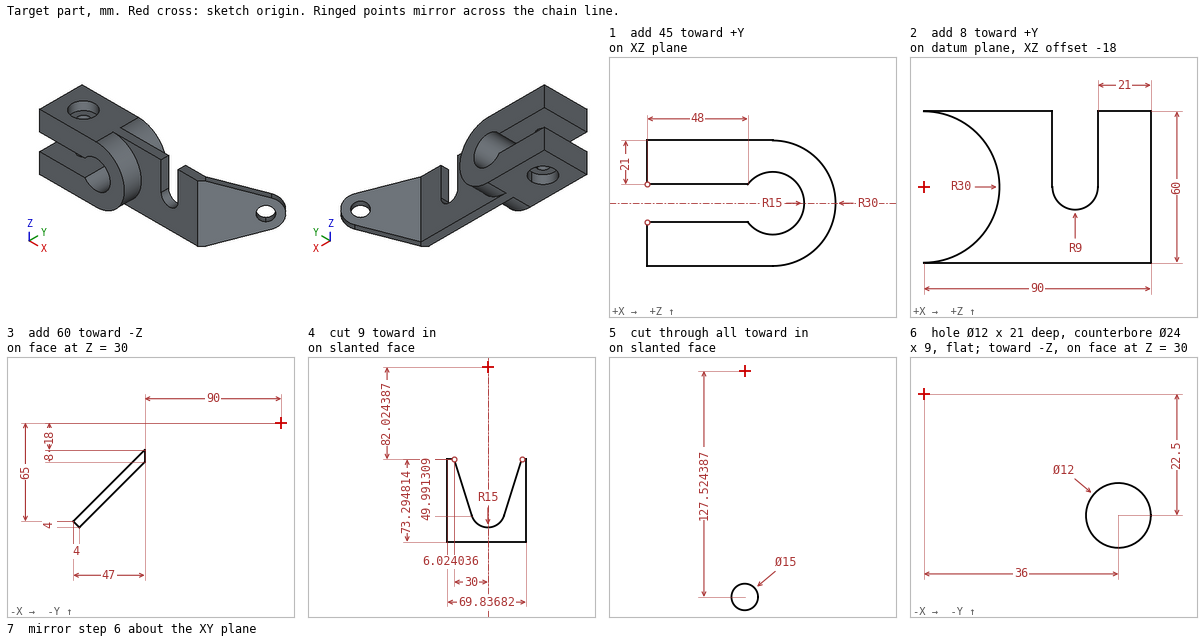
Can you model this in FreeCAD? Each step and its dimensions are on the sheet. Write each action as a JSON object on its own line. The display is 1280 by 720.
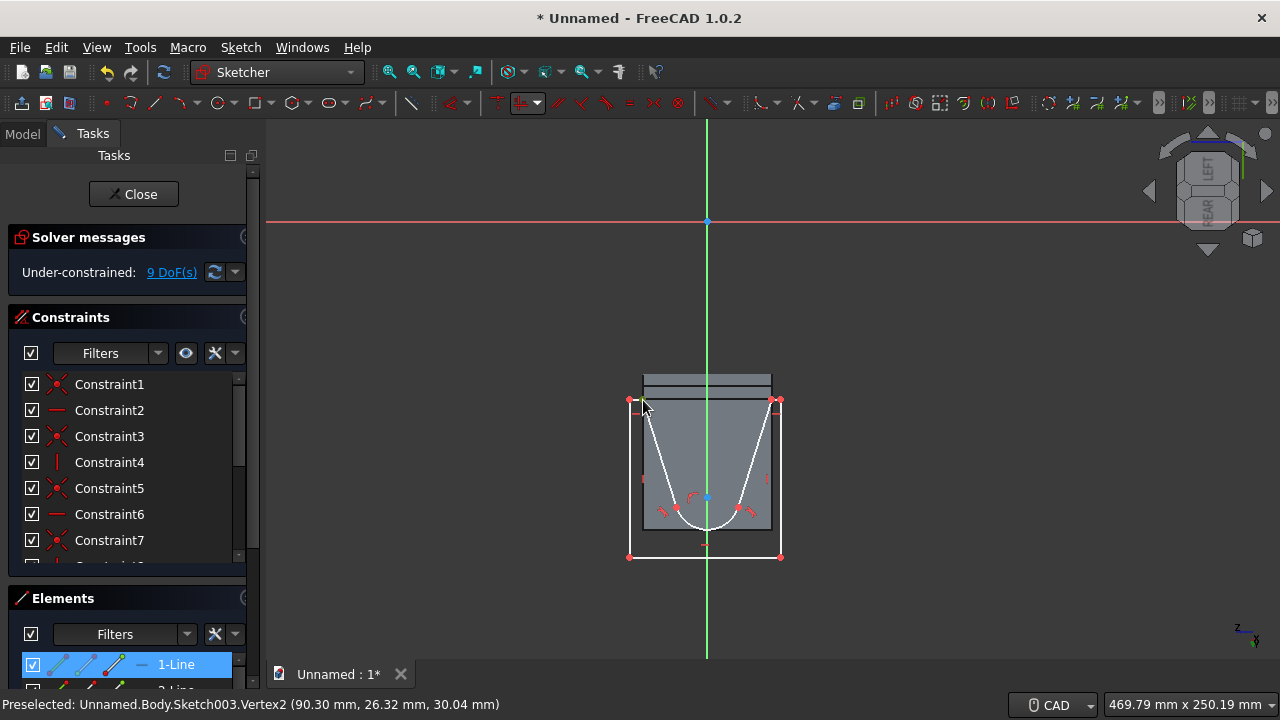
{"action": "scroll", "coordinate": [772, 400], "scroll_direction": "up", "scroll_amount": 2}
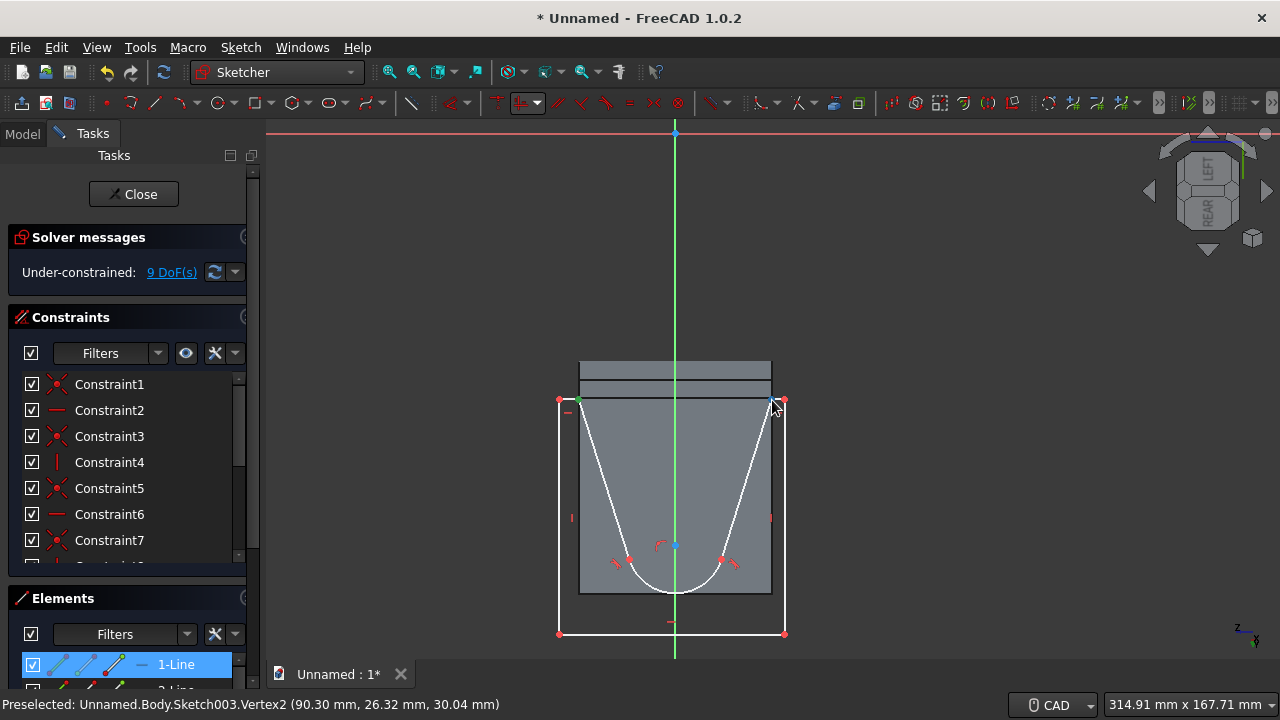
{"action": "left_click", "coordinate": [772, 399]}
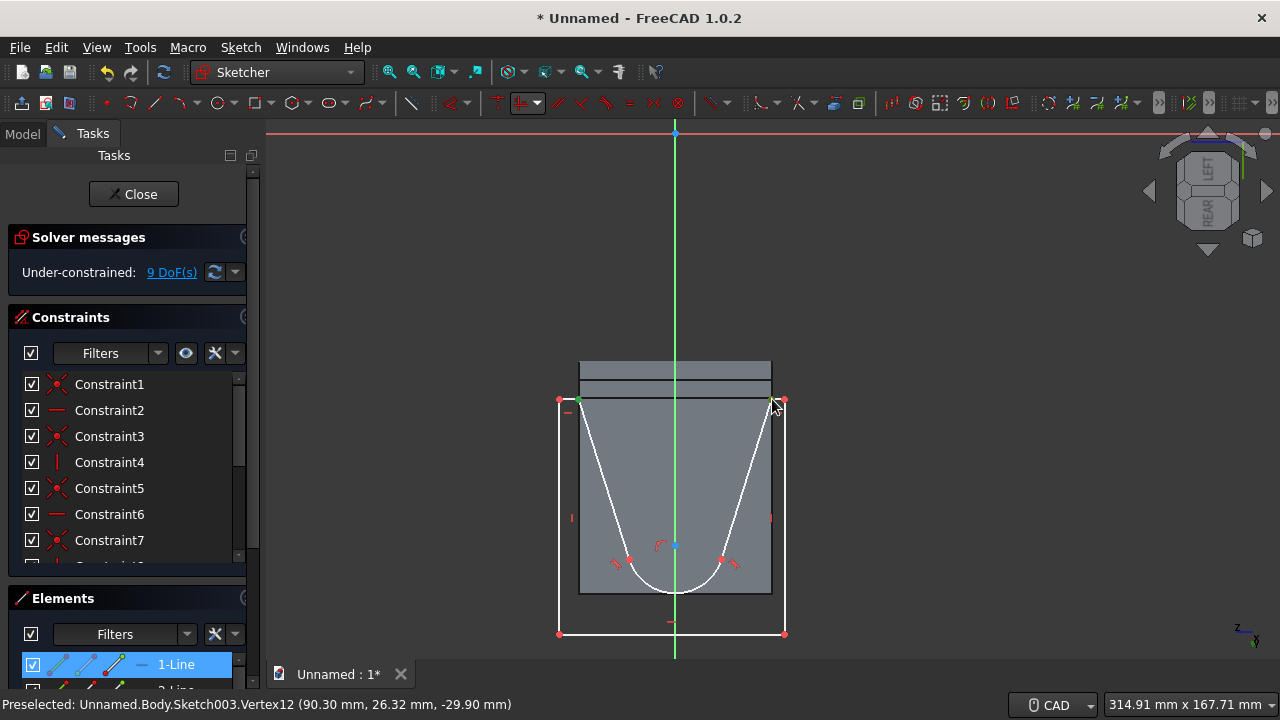
{"action": "left_click", "coordinate": [675, 562]}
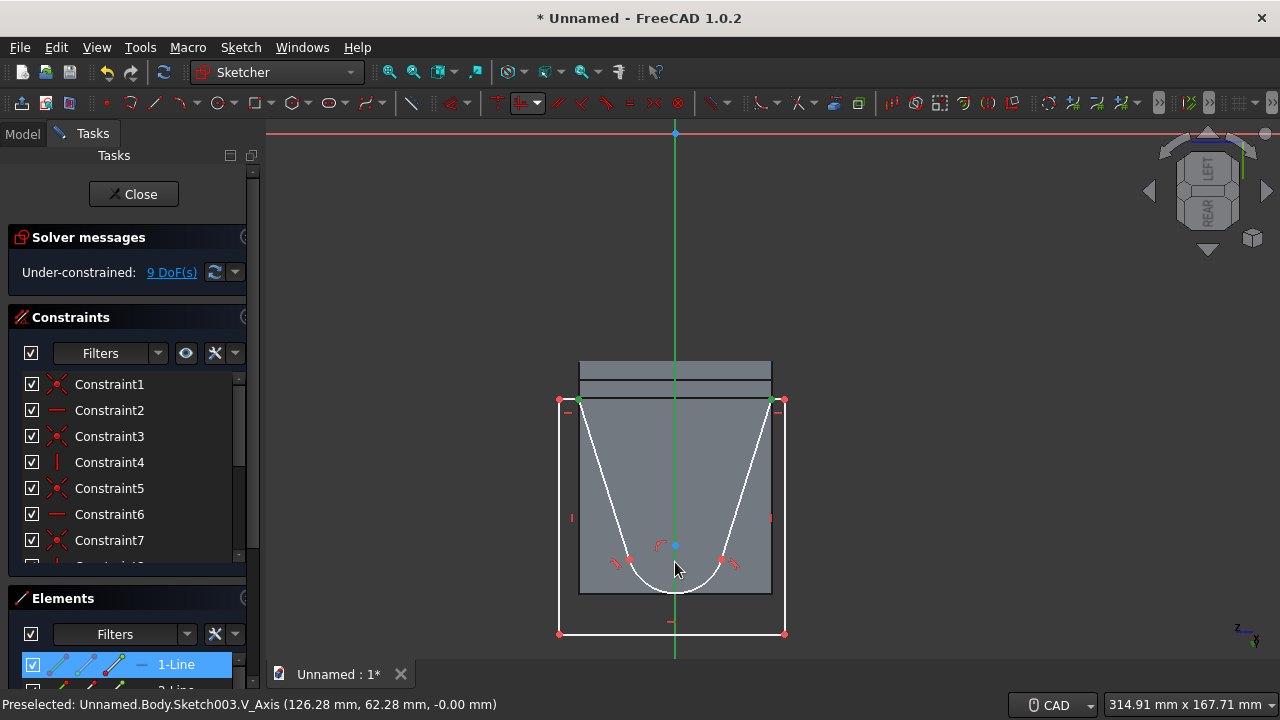
{"action": "left_click", "coordinate": [654, 104]}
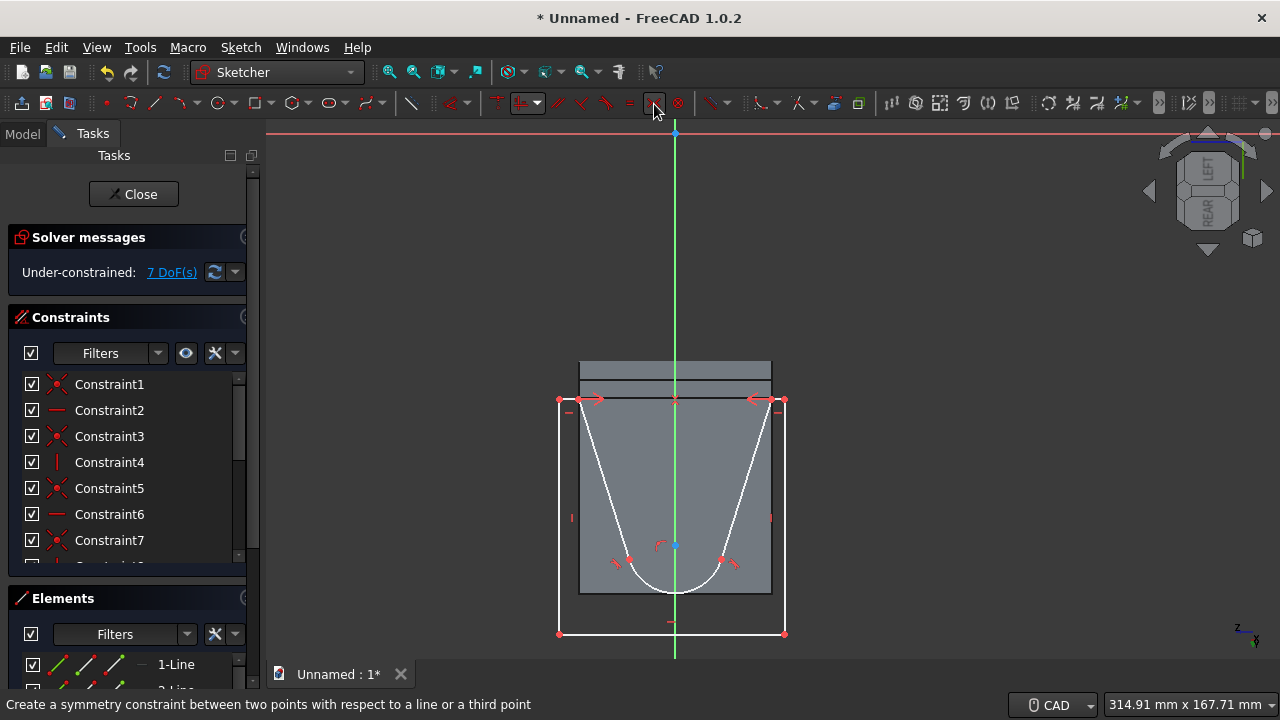
{"action": "left_click", "coordinate": [450, 104]}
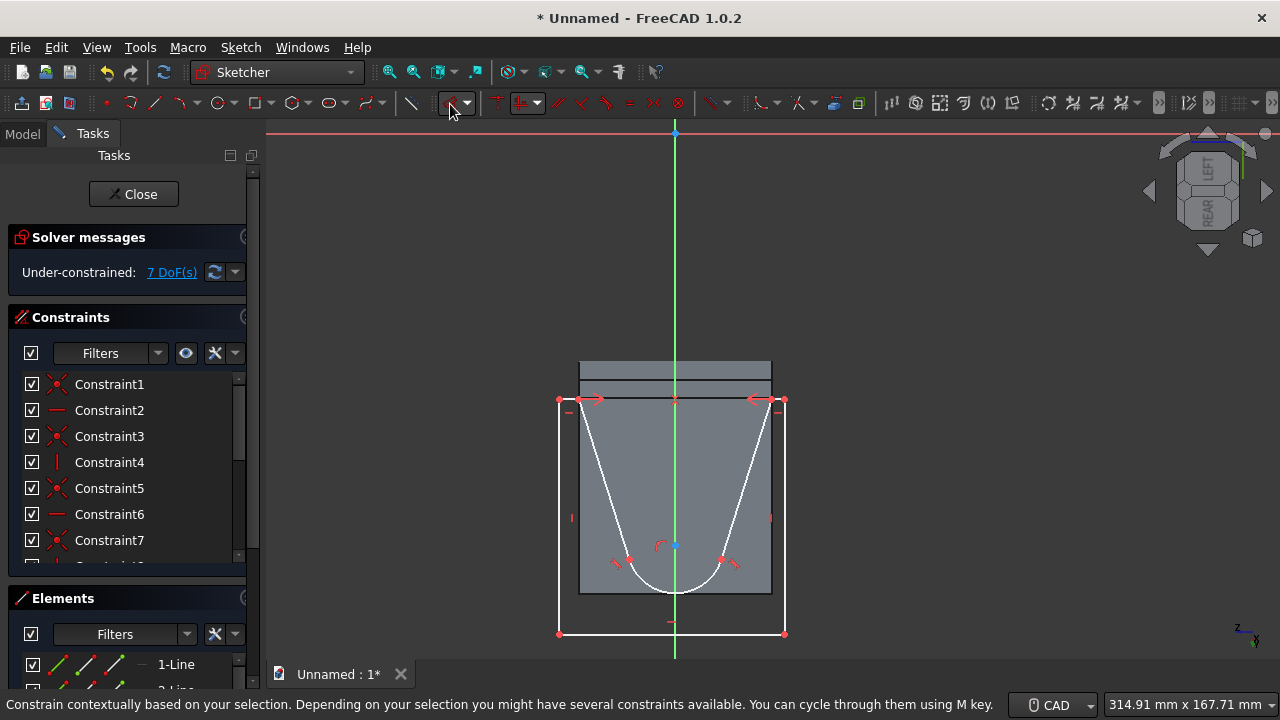
{"action": "left_click", "coordinate": [652, 587]}
{"action": "left_click", "coordinate": [636, 615]}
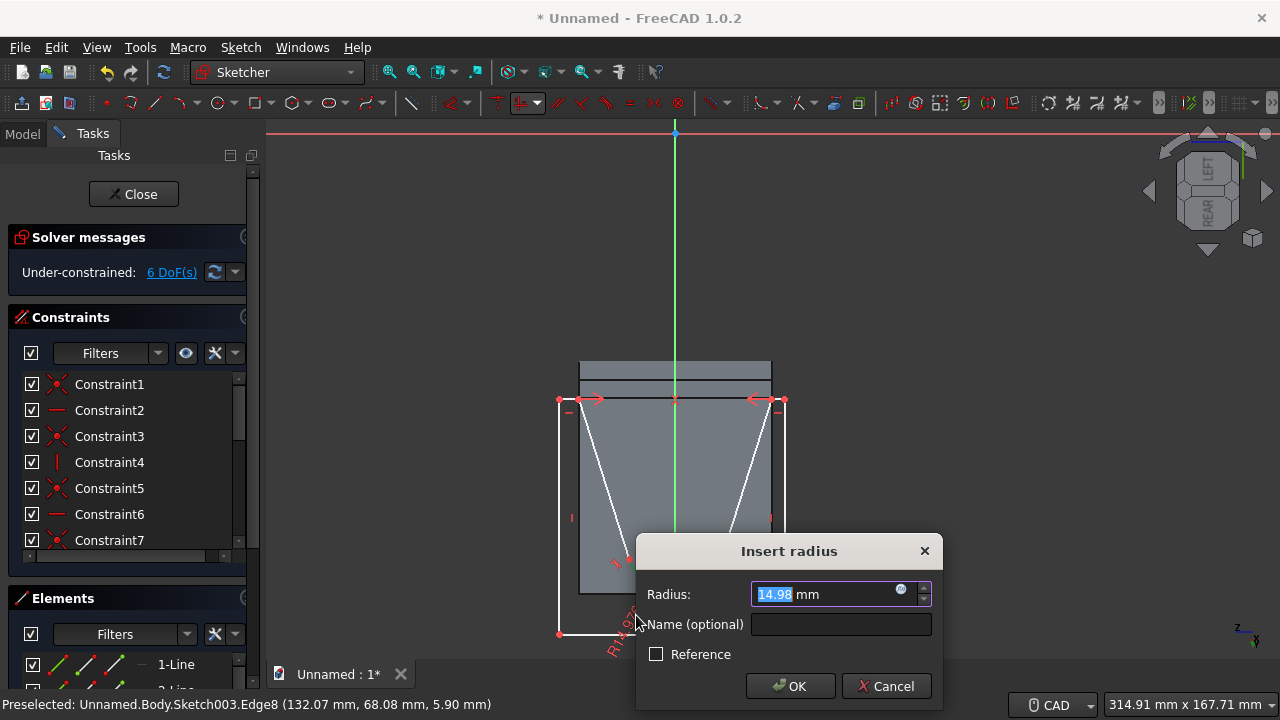
{"action": "type", "text": "15"}
{"action": "key", "text": "Return"}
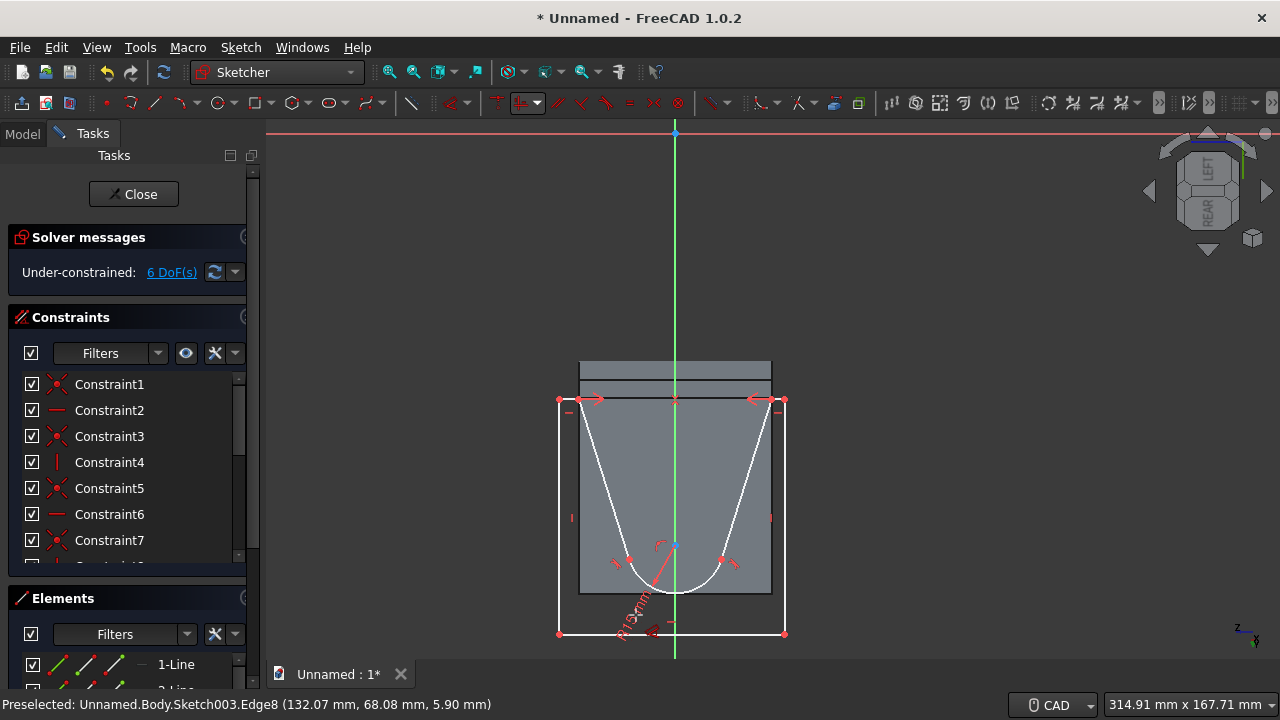
{"action": "left_click", "coordinate": [579, 399]}
{"action": "left_click", "coordinate": [627, 433]}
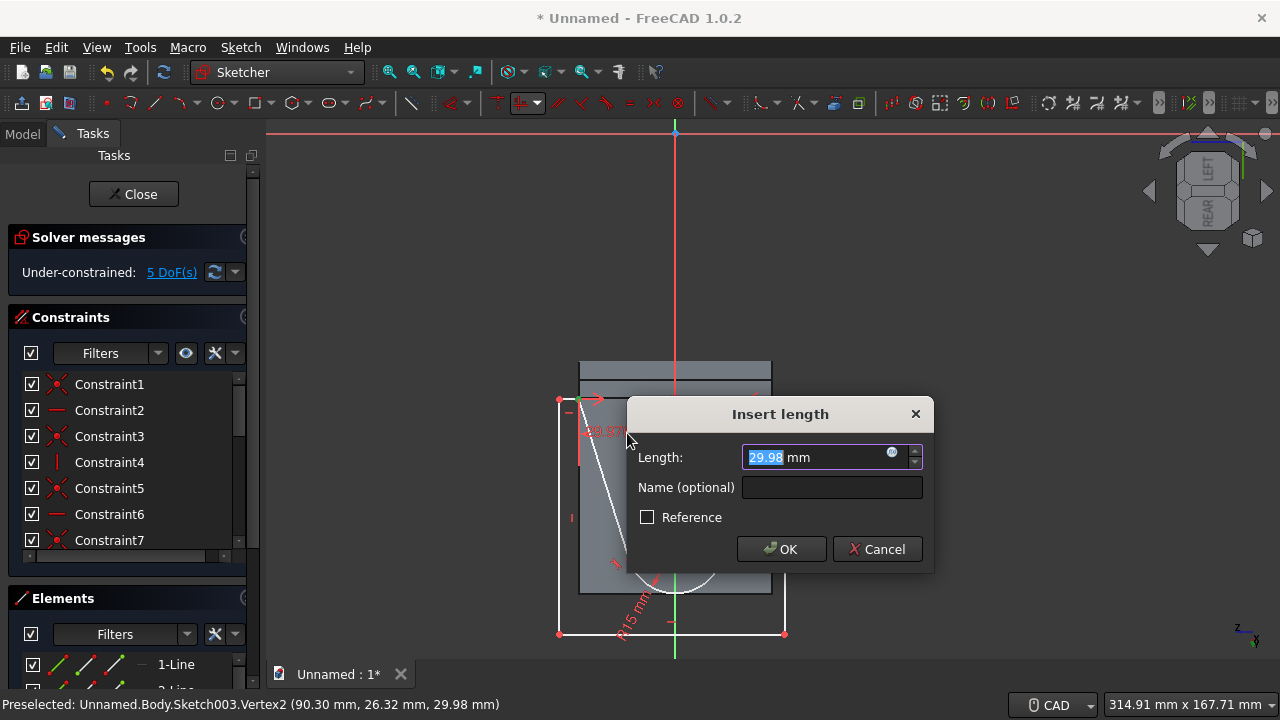
{"action": "type", "text": "30"}
{"action": "key", "text": "Return"}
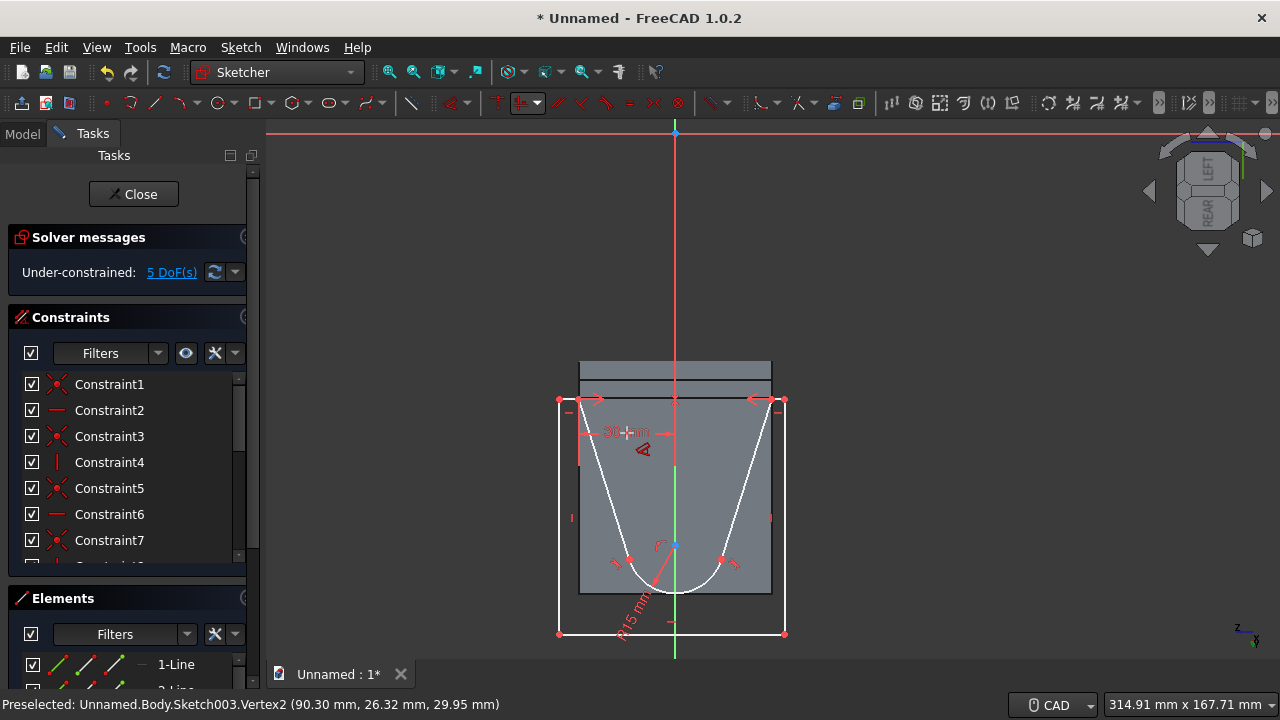
{"action": "scroll", "coordinate": [569, 399], "scroll_direction": "up", "scroll_amount": 4}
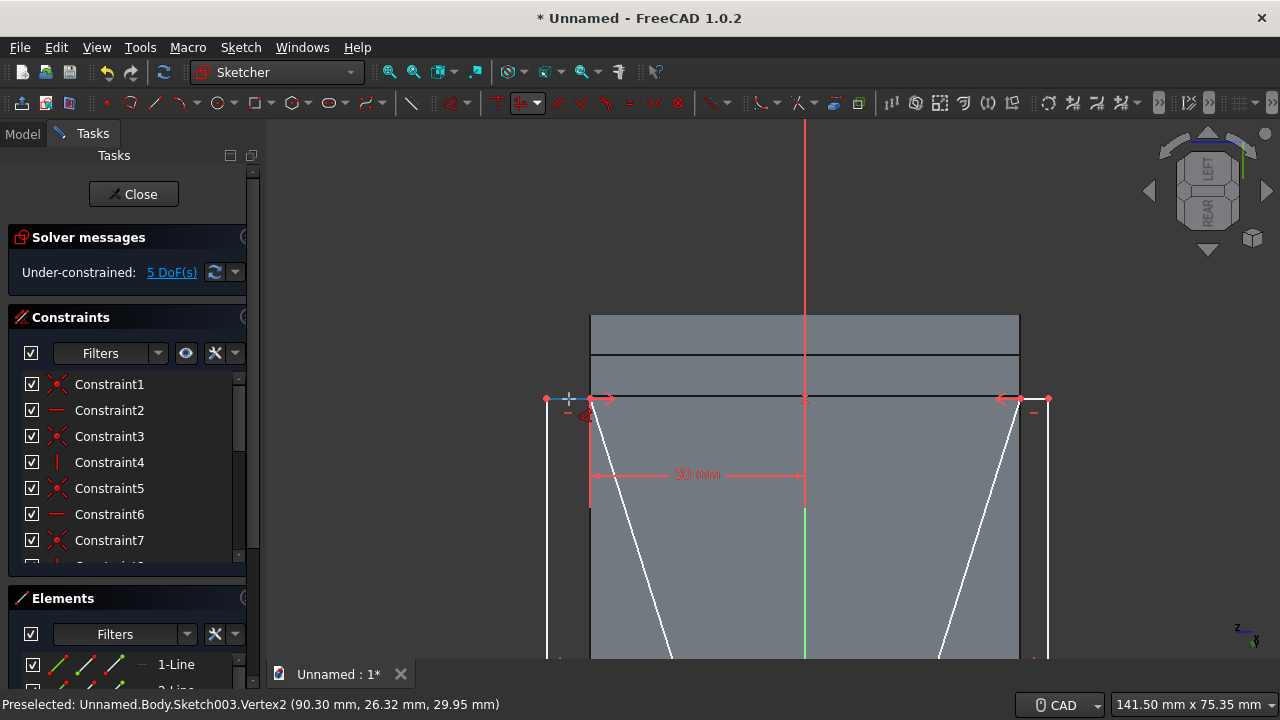
{"action": "left_click", "coordinate": [569, 399]}
{"action": "left_click", "coordinate": [569, 433]}